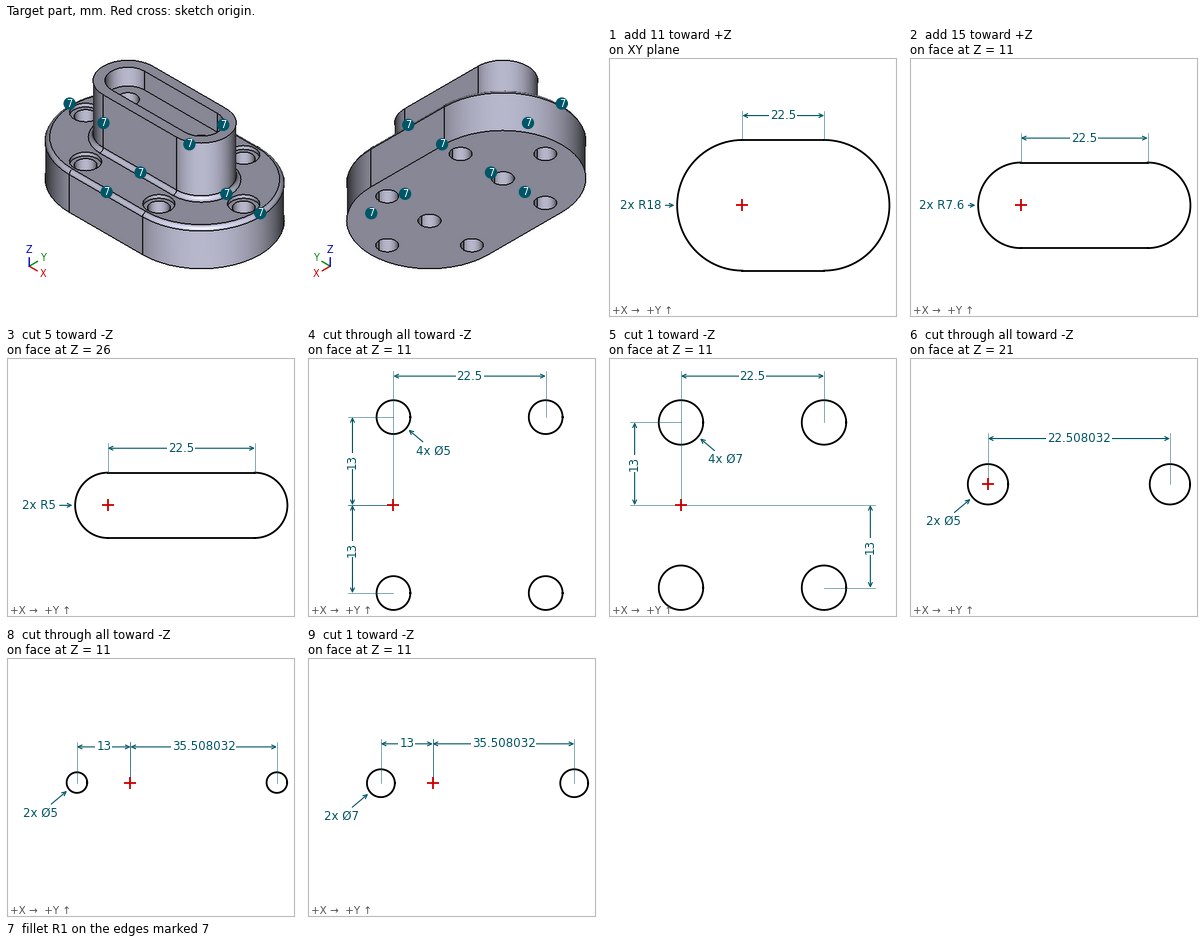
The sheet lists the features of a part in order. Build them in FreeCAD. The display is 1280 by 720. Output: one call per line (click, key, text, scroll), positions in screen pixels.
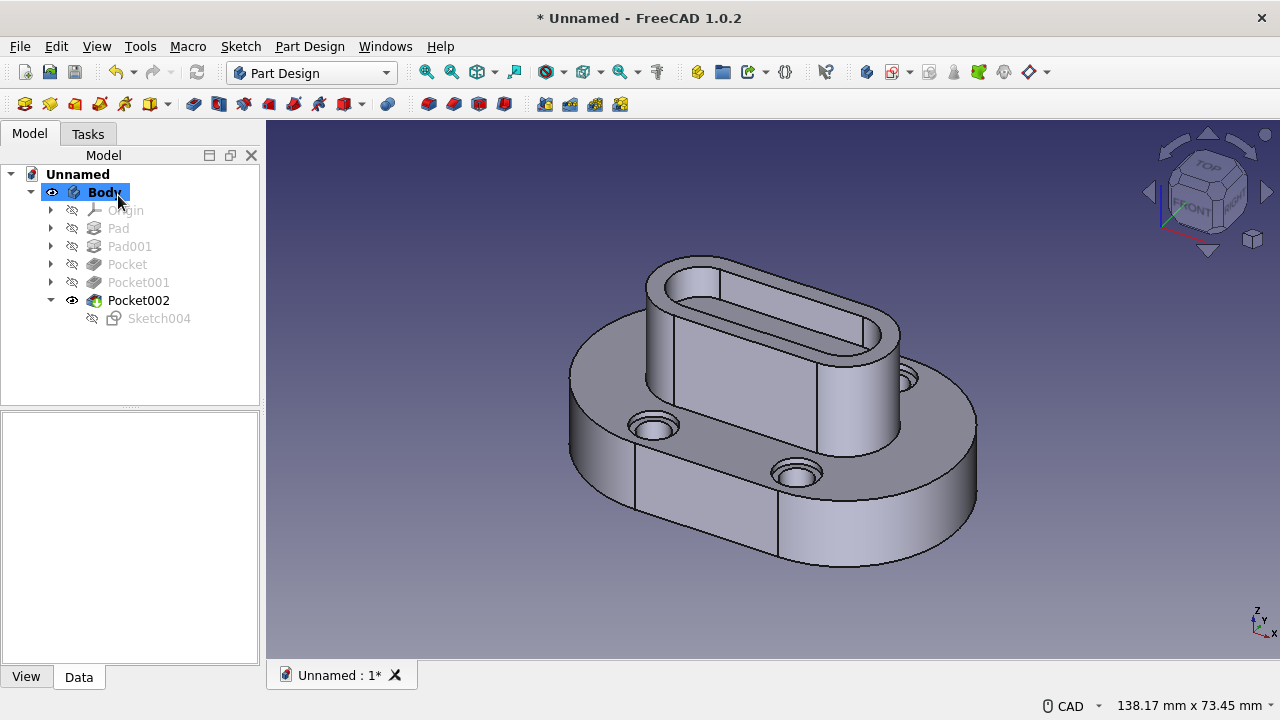
key(0)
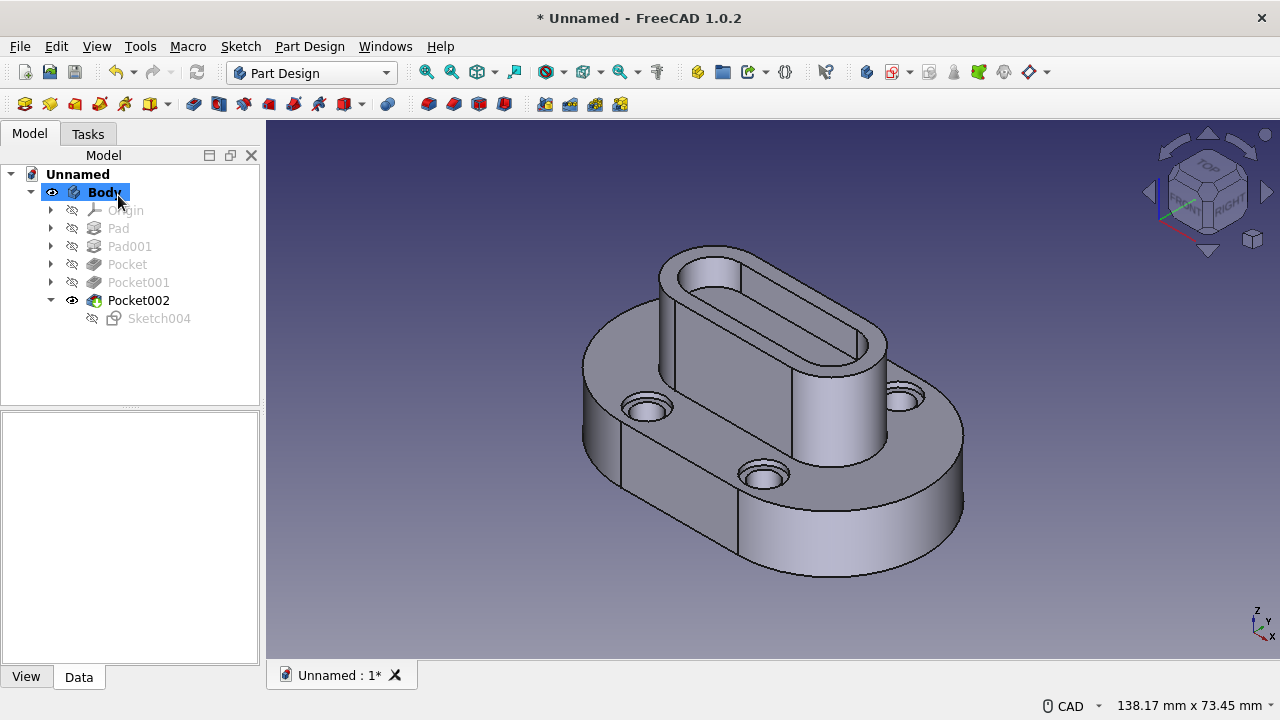
key(2)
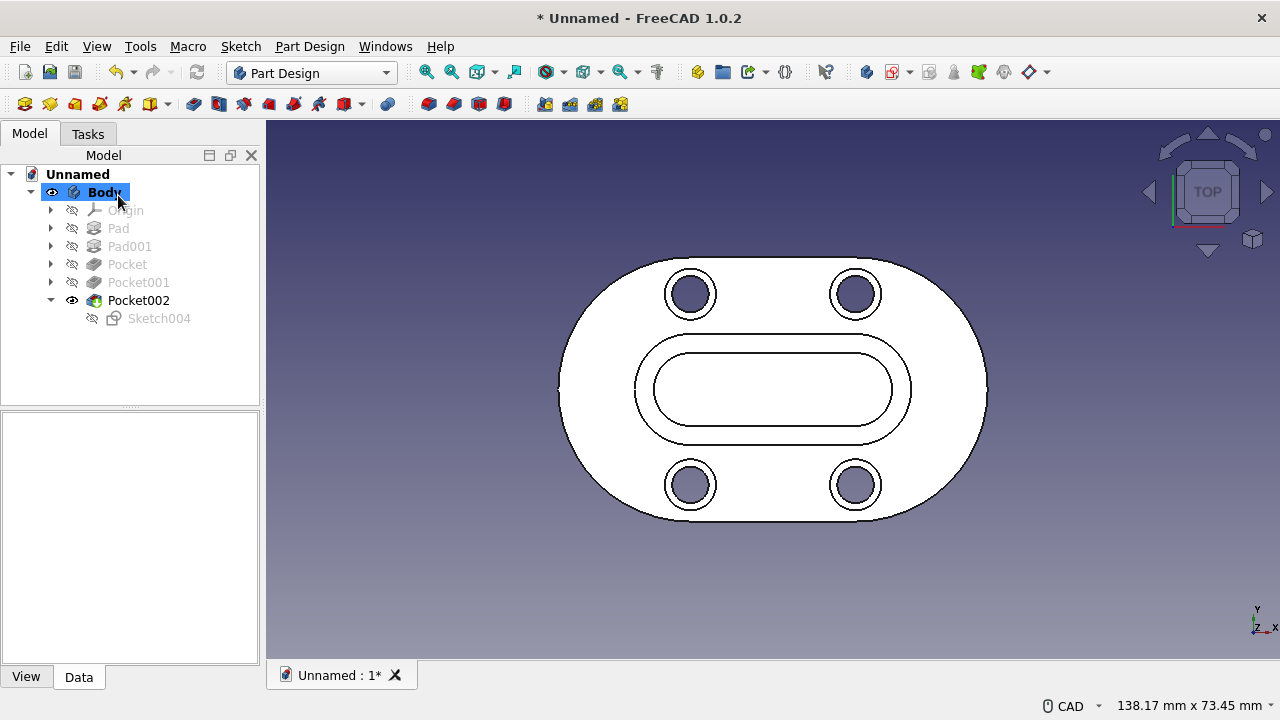
click(841, 389)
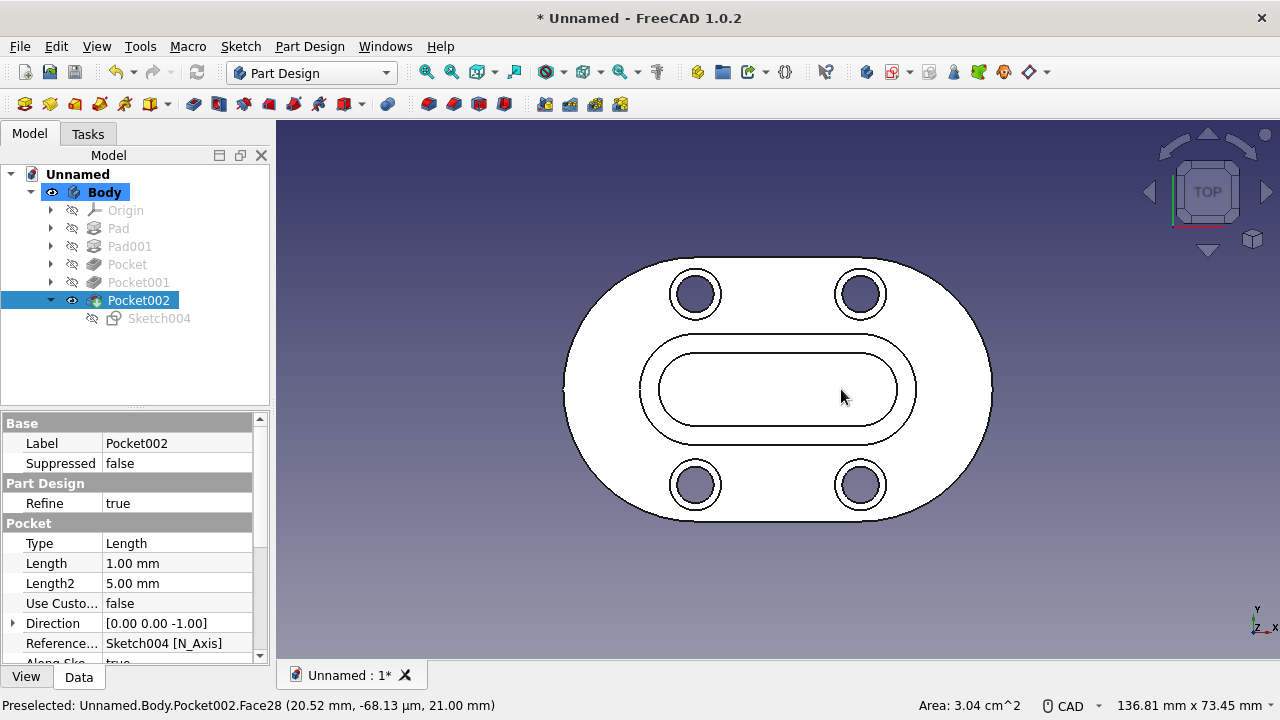
click(892, 72)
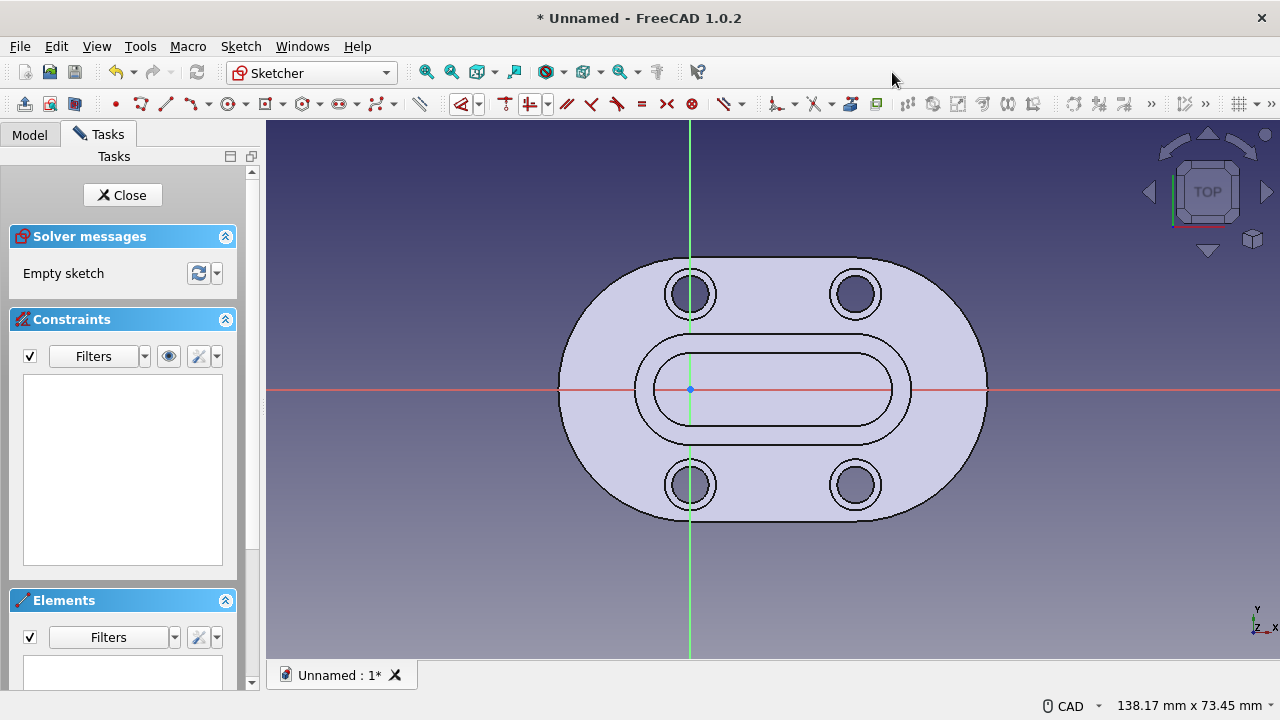
key(q)
key(s)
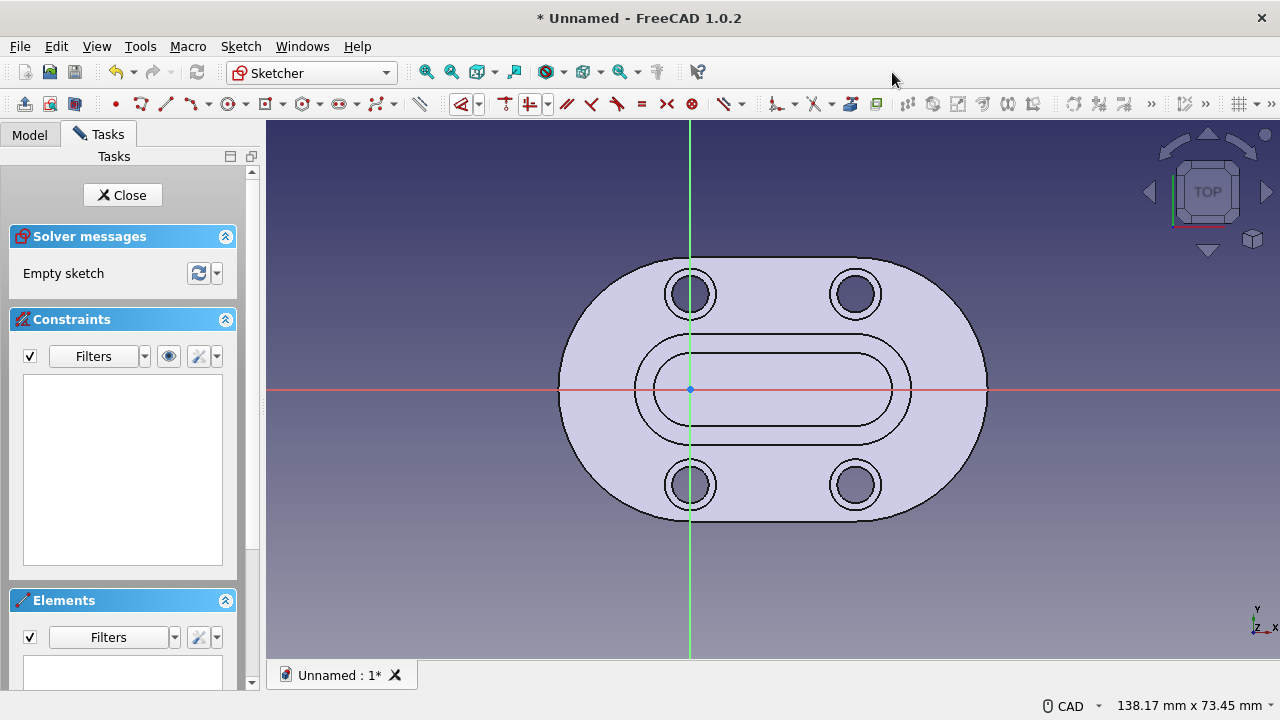
scroll(813, 390, up, 5)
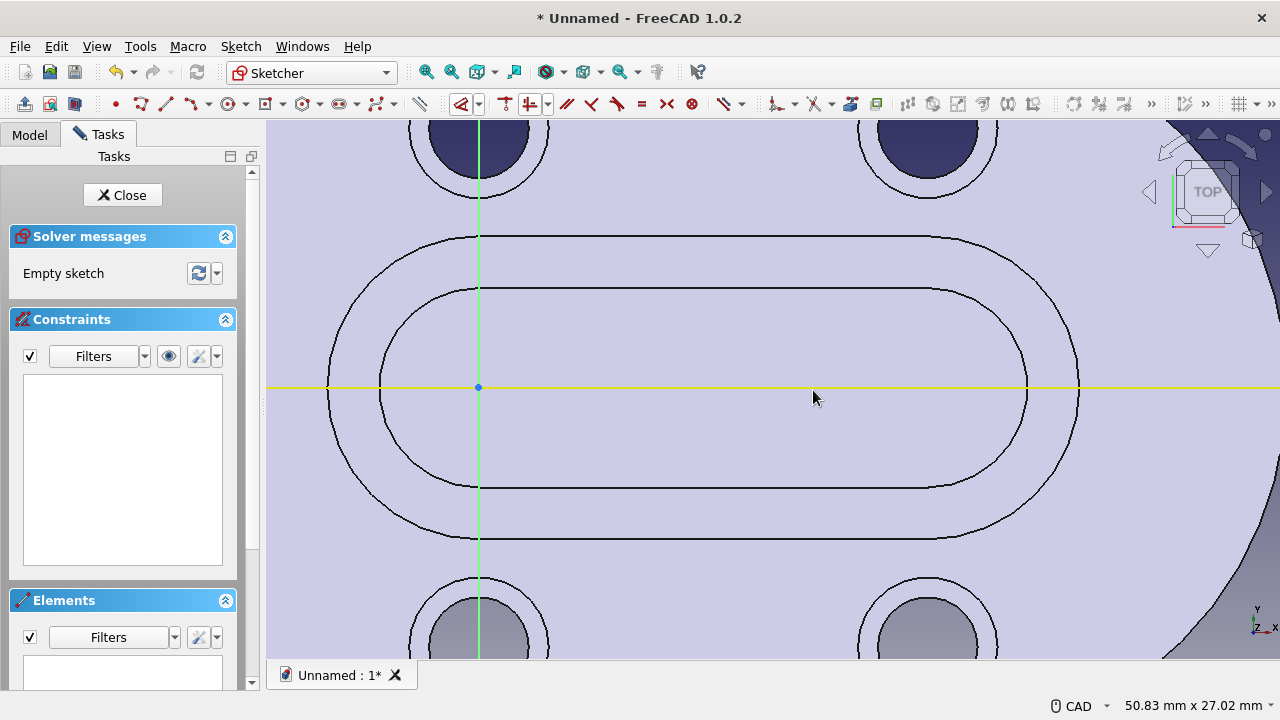
key(g)
key(c)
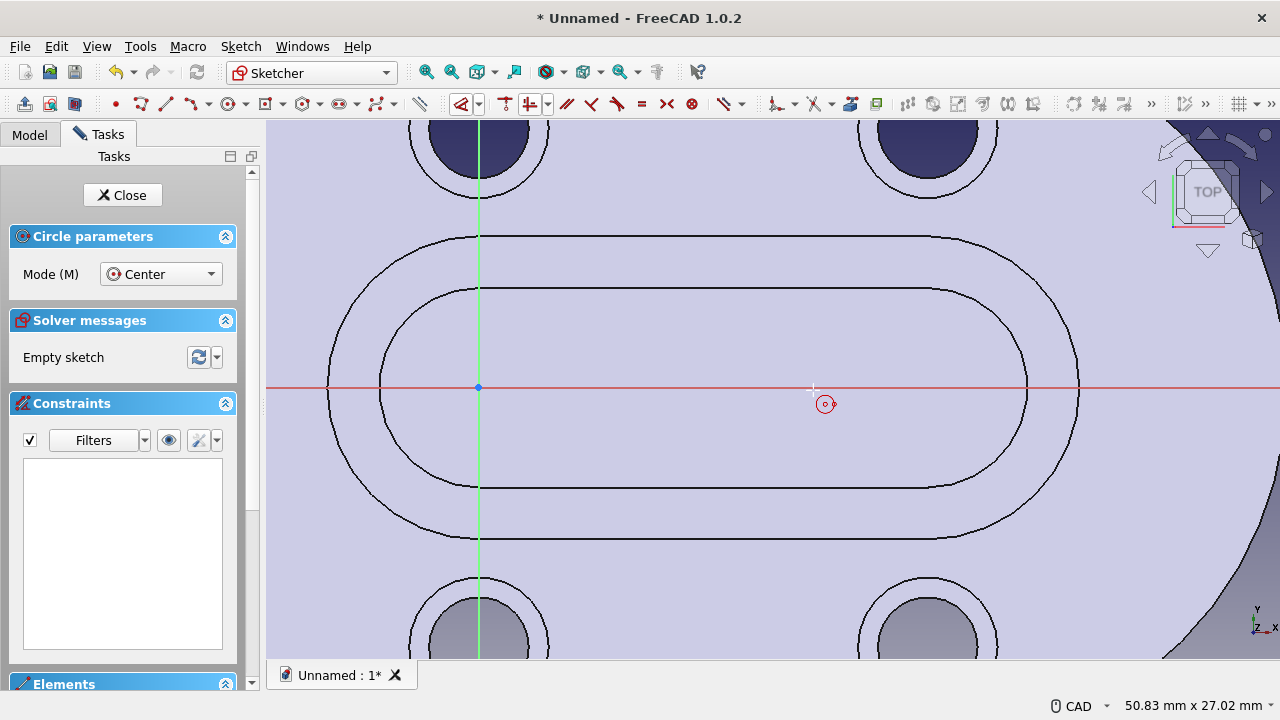
click(479, 388)
move(514, 353)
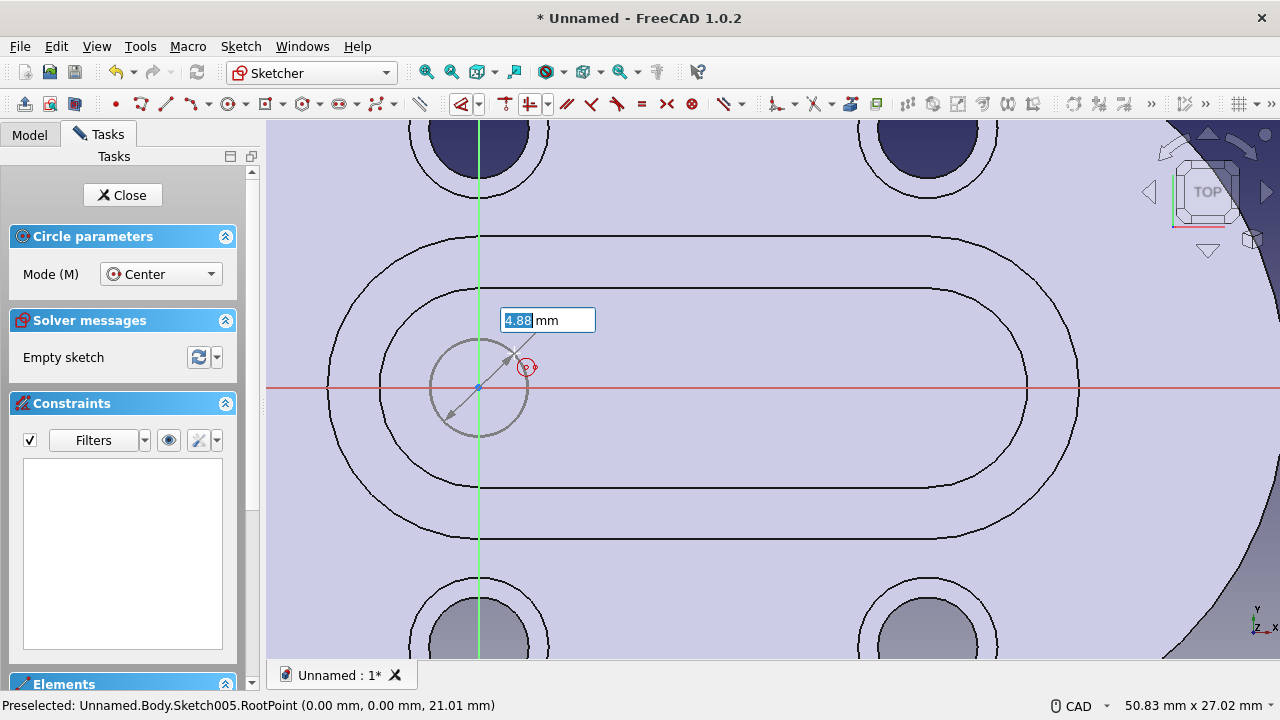
text(5)
key(Return)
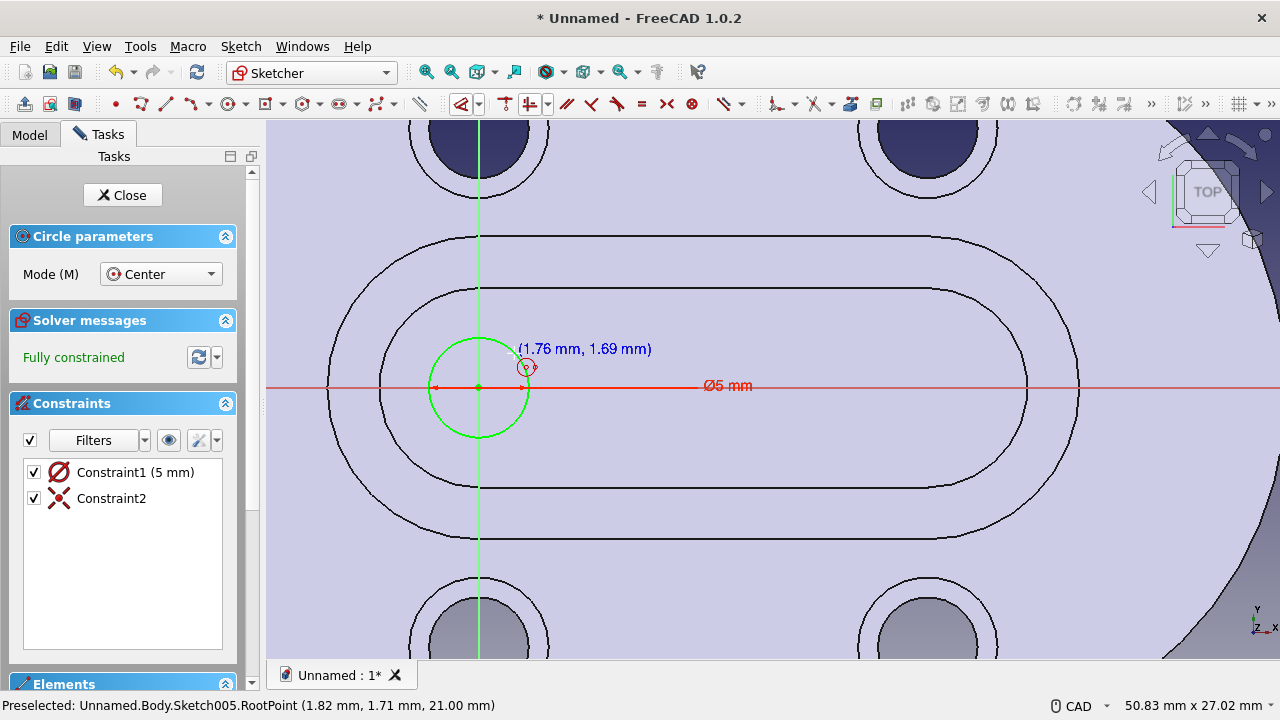
click(928, 388)
move(963, 353)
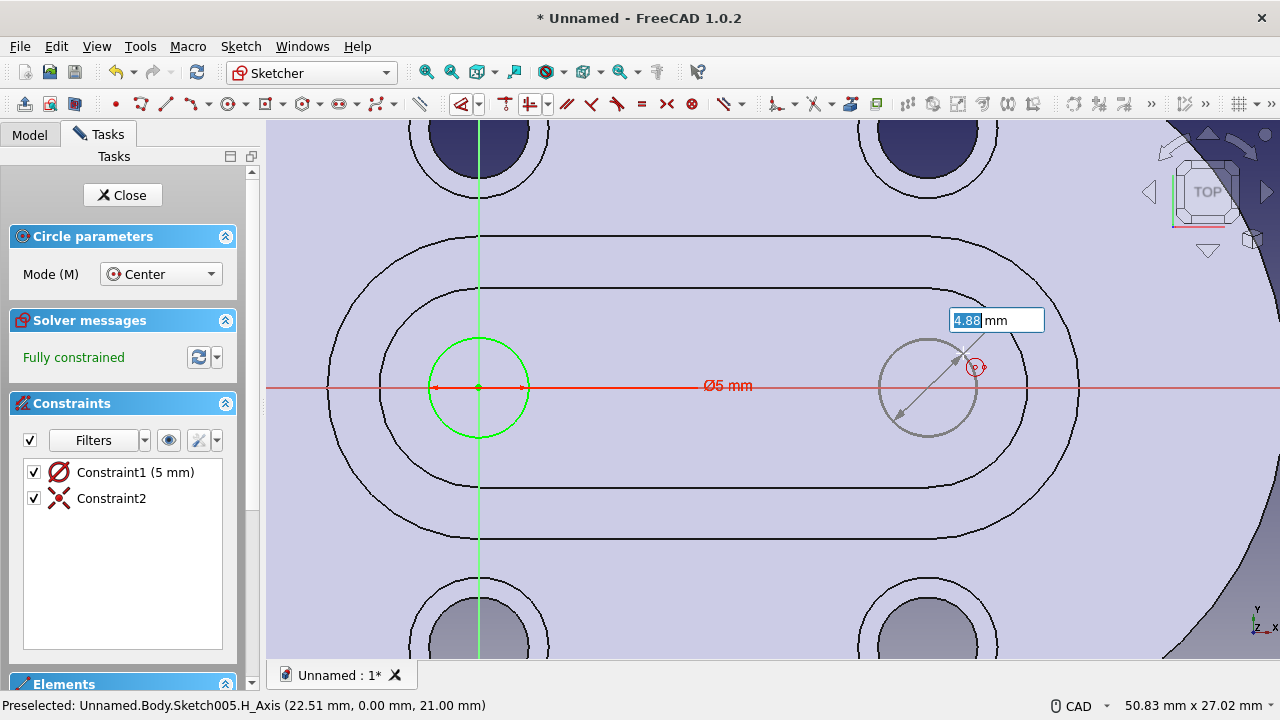
text(5)
key(Return)
key(Escape)